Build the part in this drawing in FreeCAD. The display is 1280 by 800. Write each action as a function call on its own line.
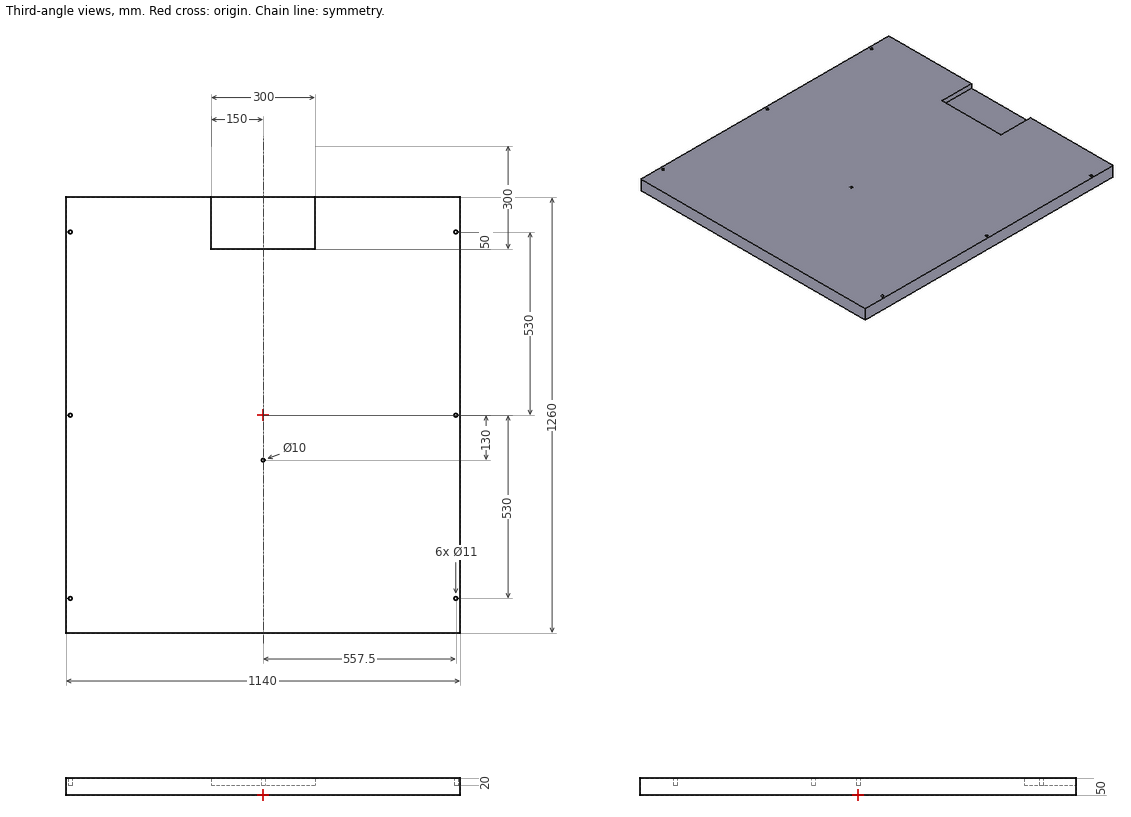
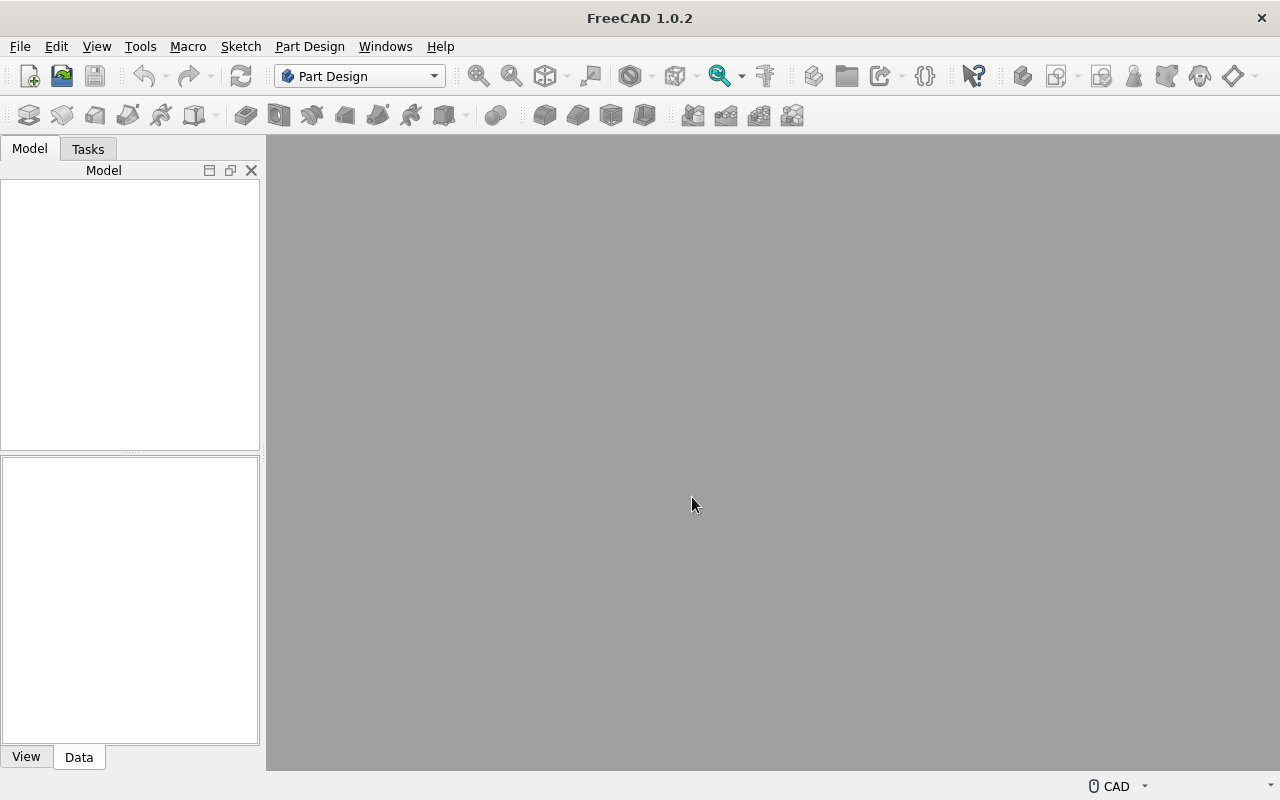
click(29, 76)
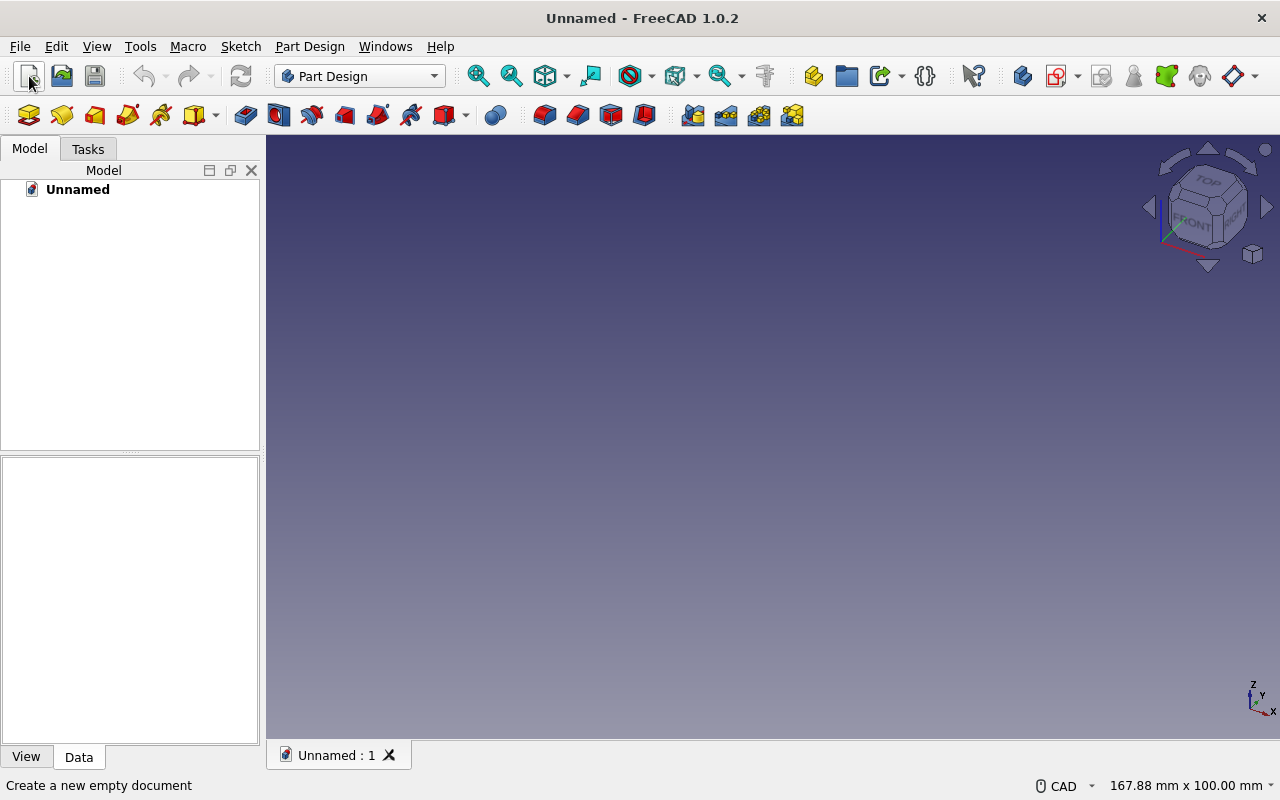
click(1056, 76)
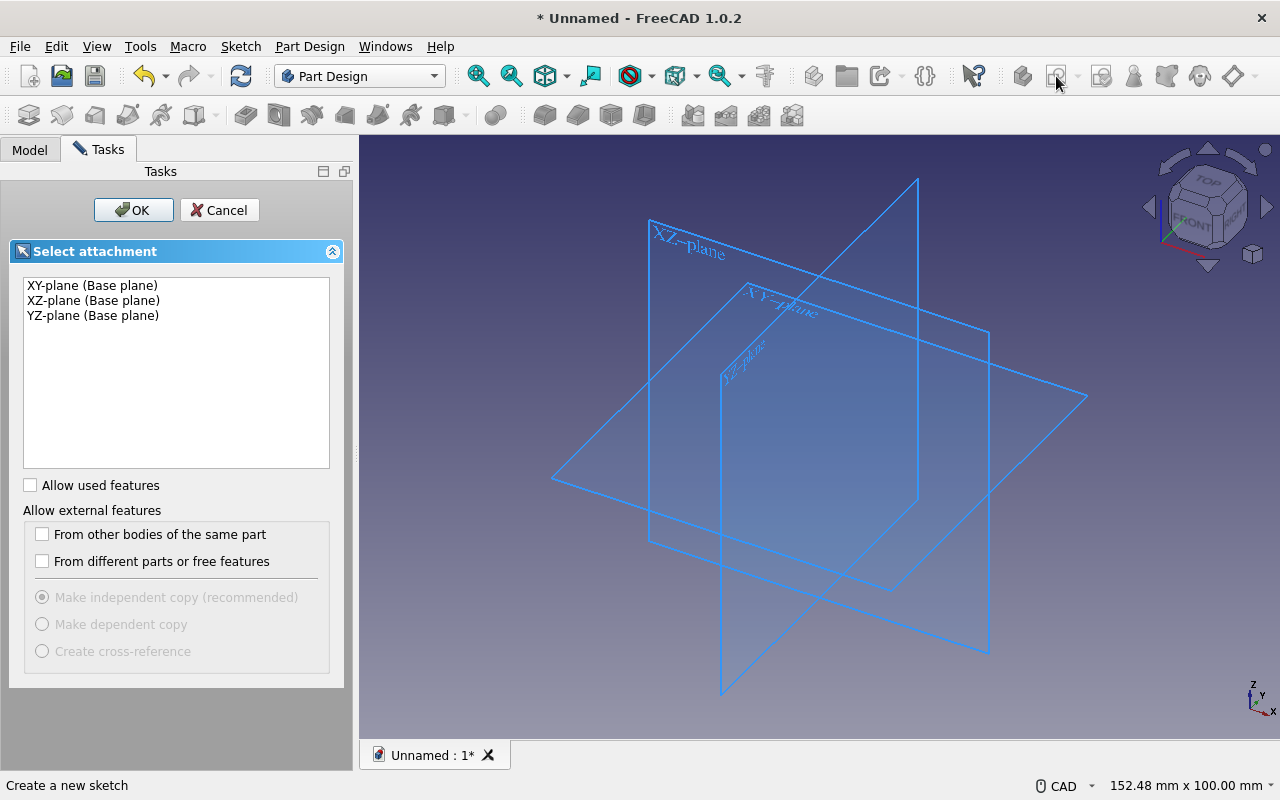
click(84, 286)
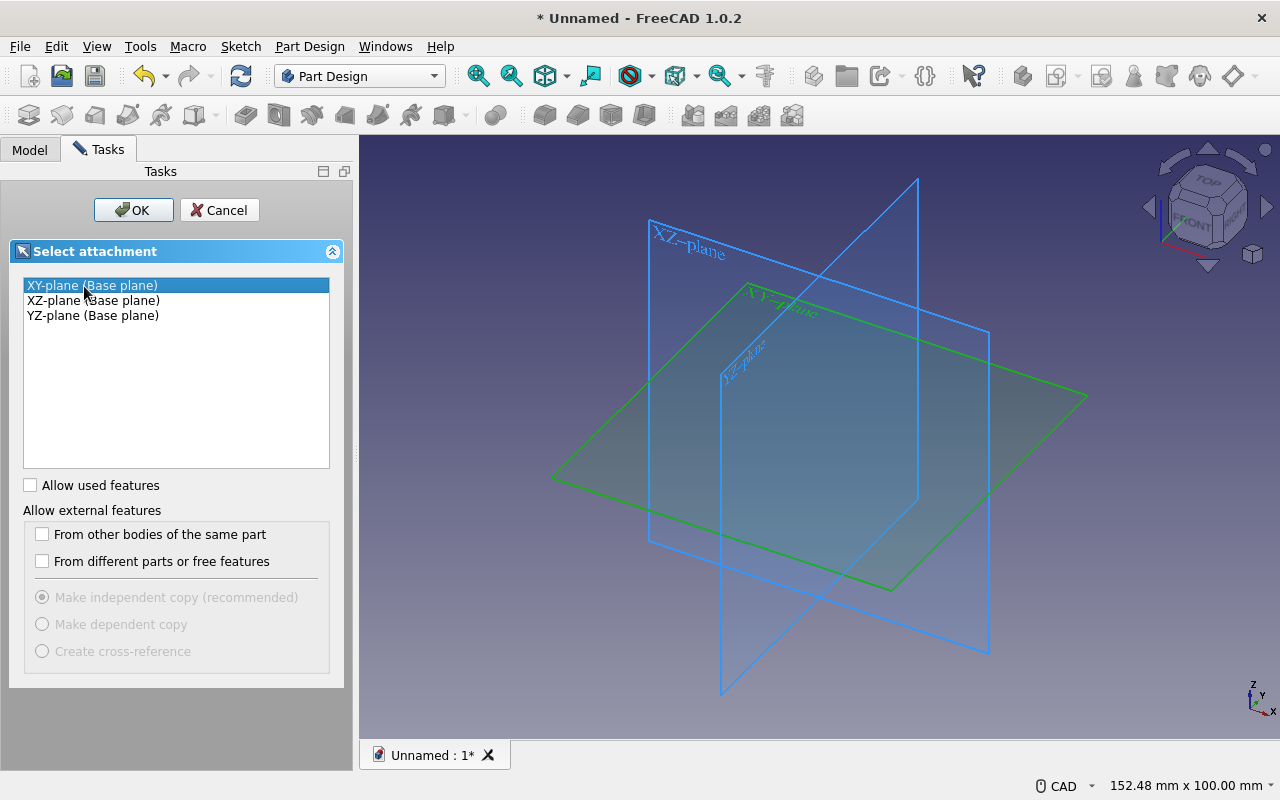
click(134, 210)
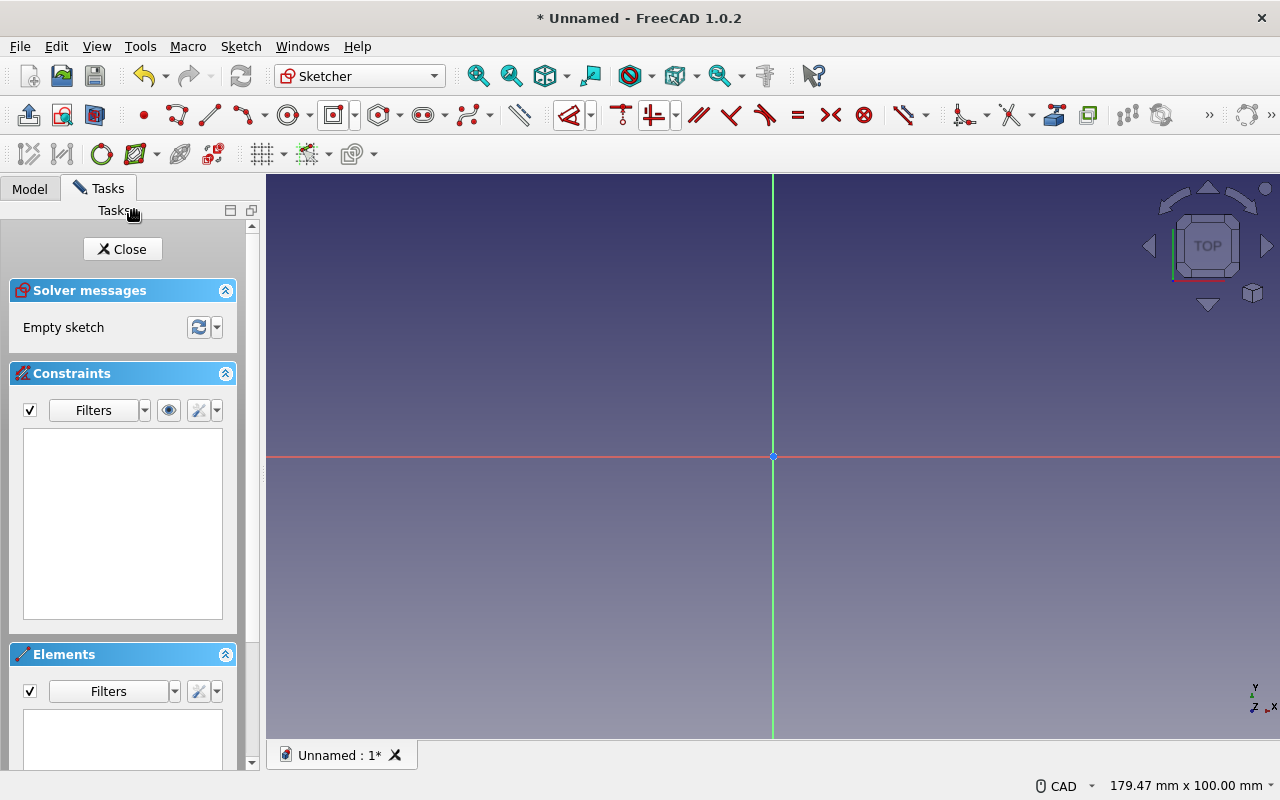
scroll(701, 457, down, 15)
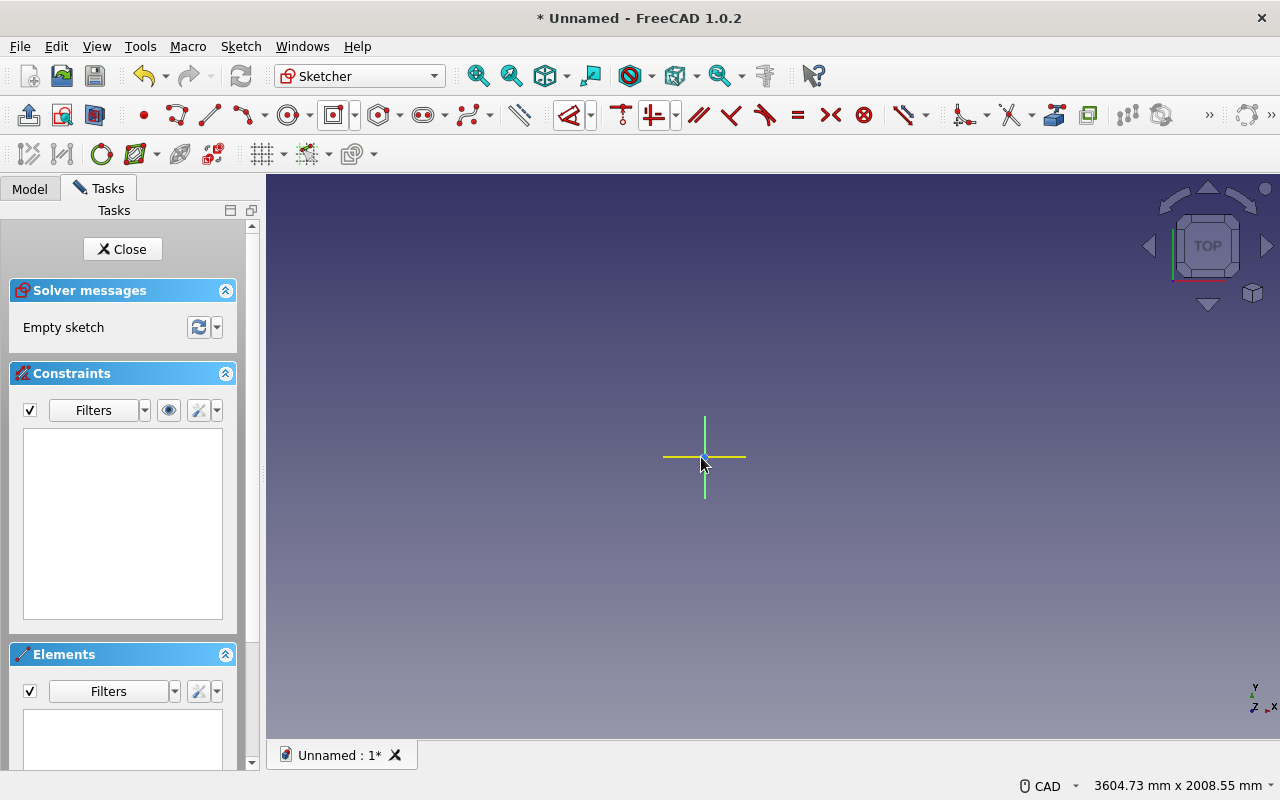
click(332, 116)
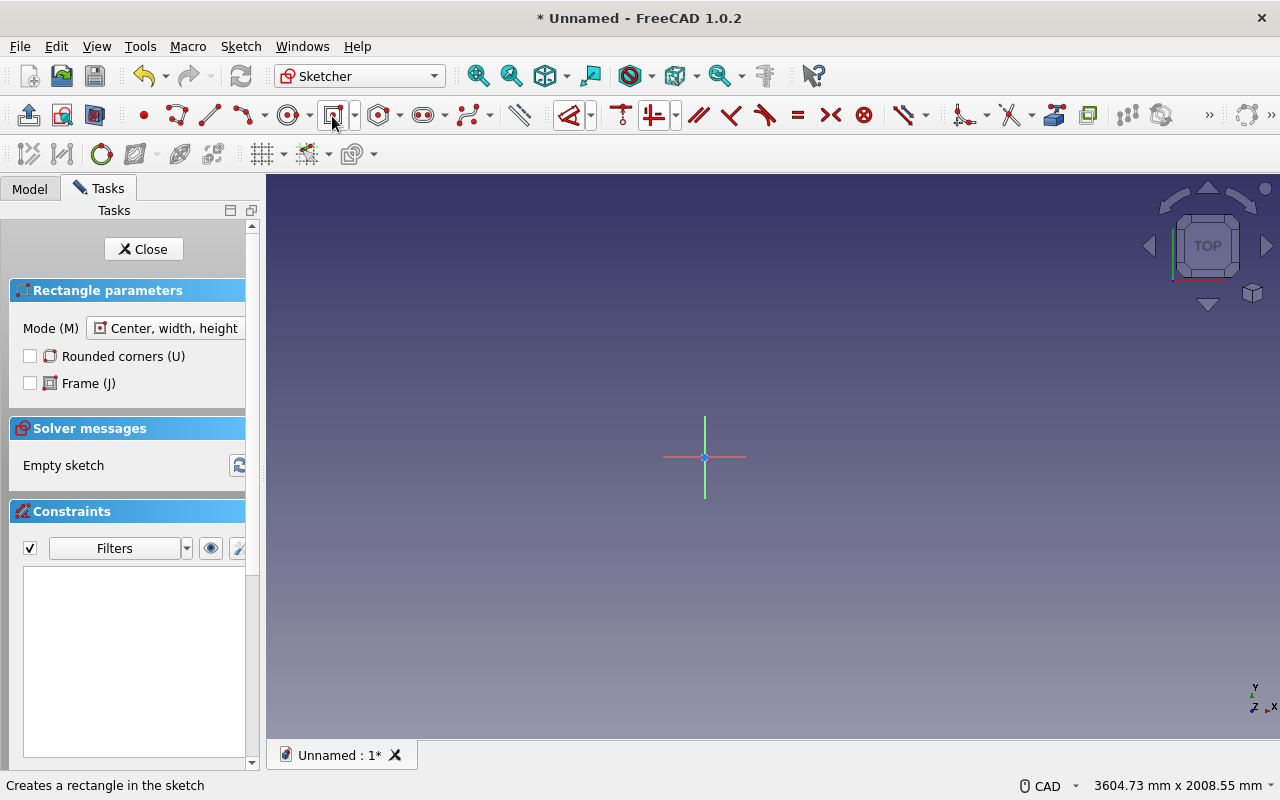
click(705, 457)
move(865, 280)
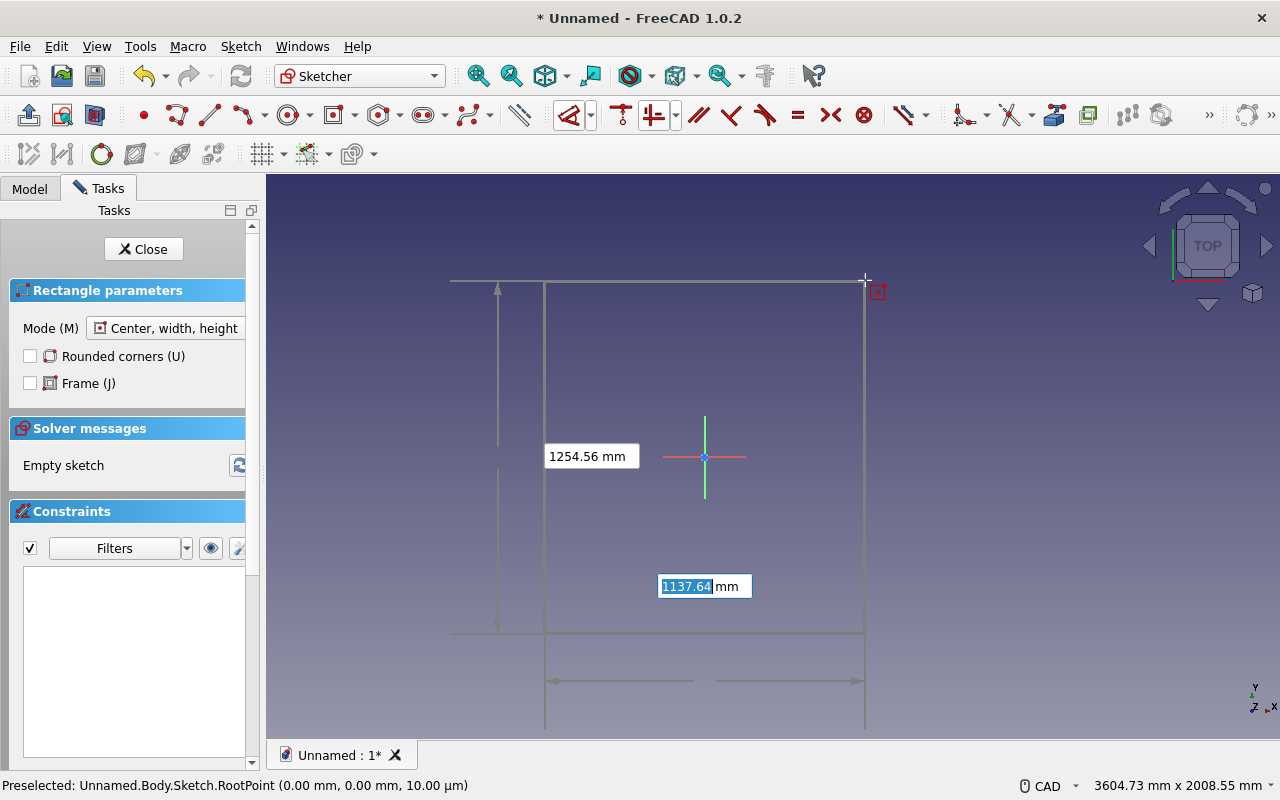
text(1140)
key(Tab)
text(1260)
key(Return)
key(Escape)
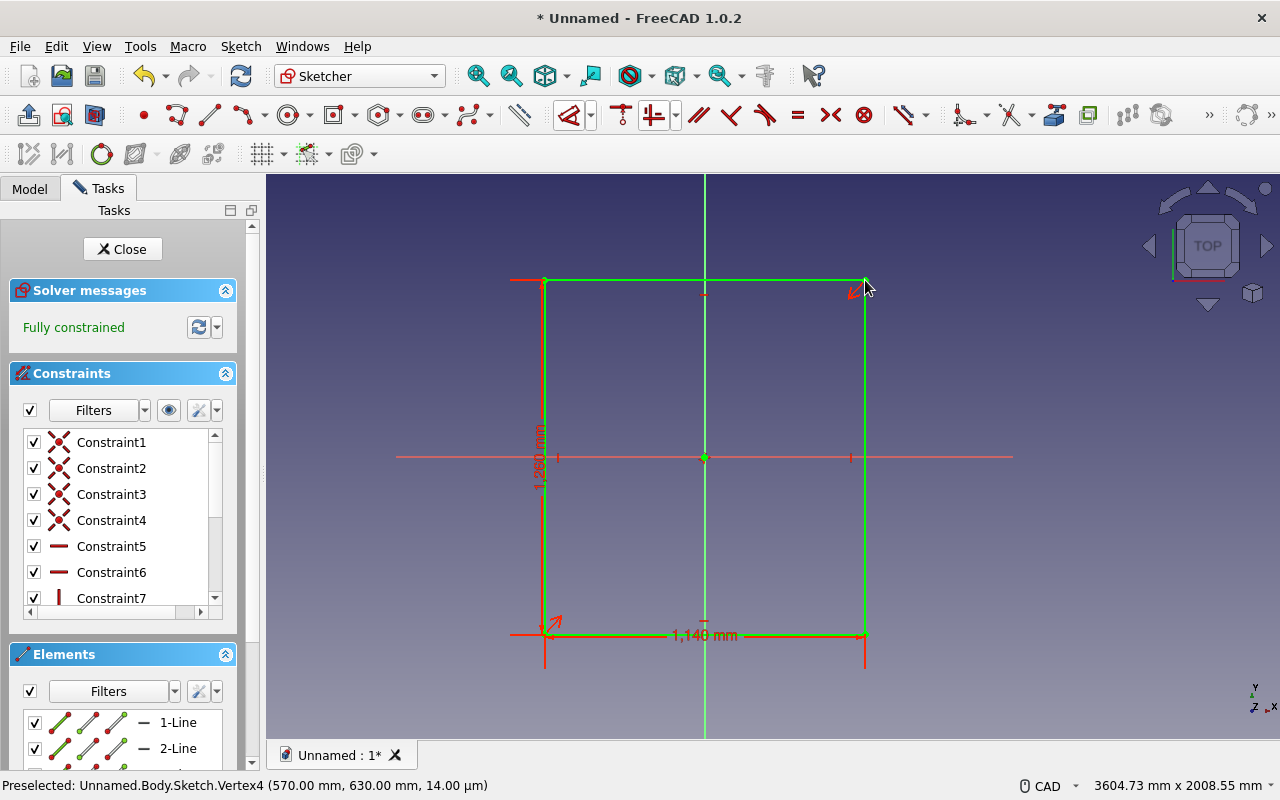
click(123, 249)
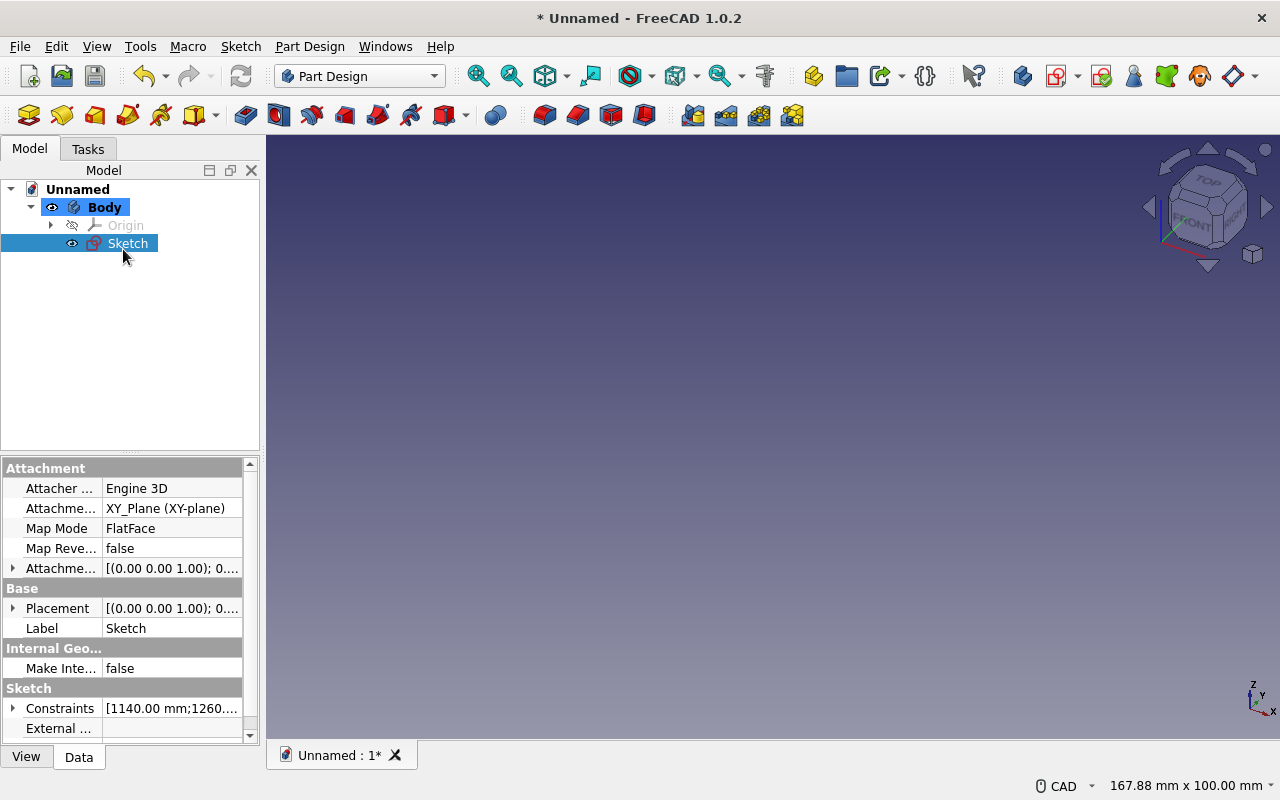
click(29, 116)